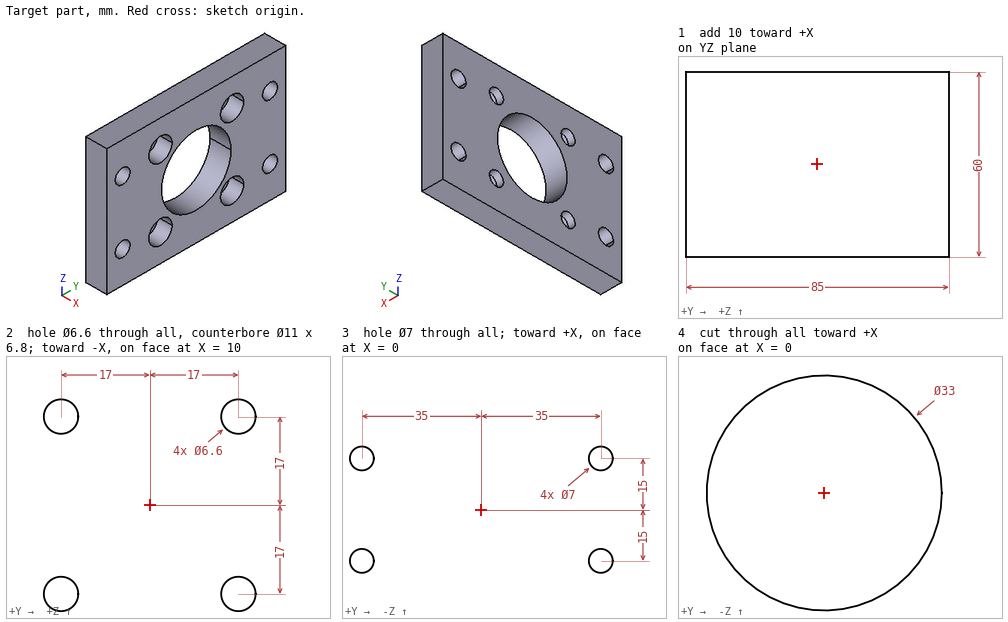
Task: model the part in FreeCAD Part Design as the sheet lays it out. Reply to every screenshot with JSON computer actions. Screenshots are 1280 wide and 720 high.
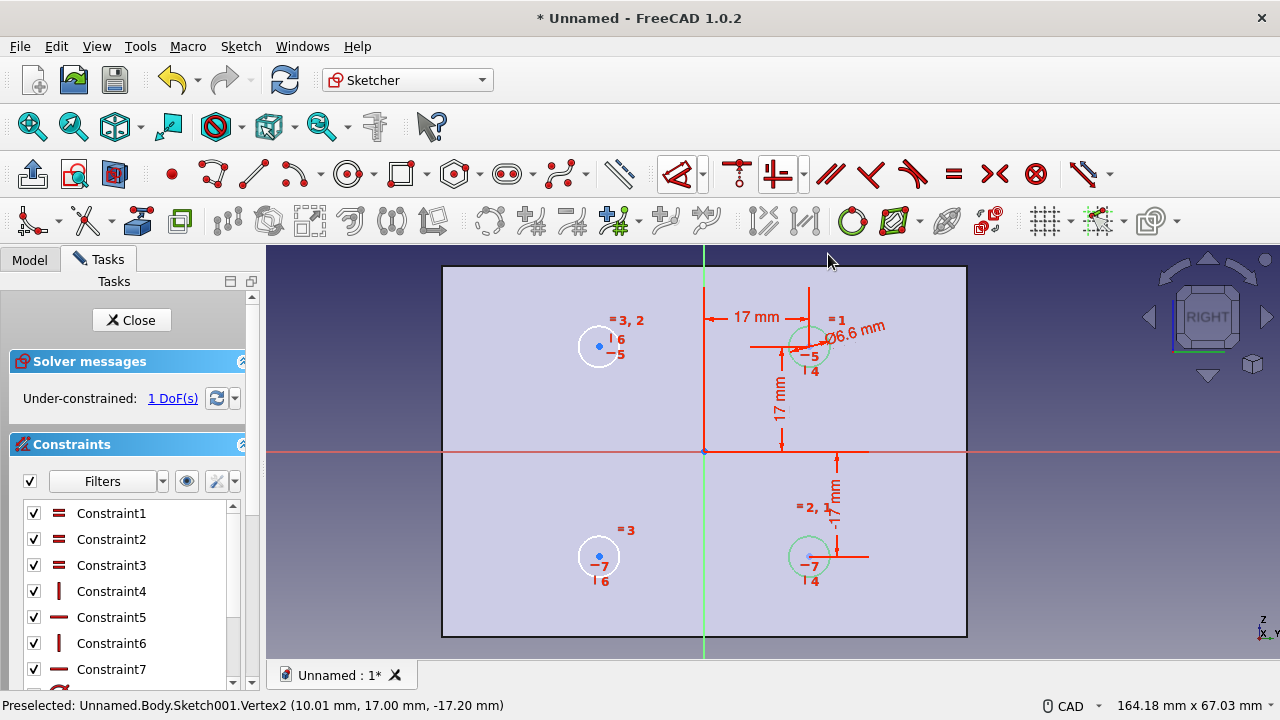
{"action": "left_click", "coordinate": [599, 347]}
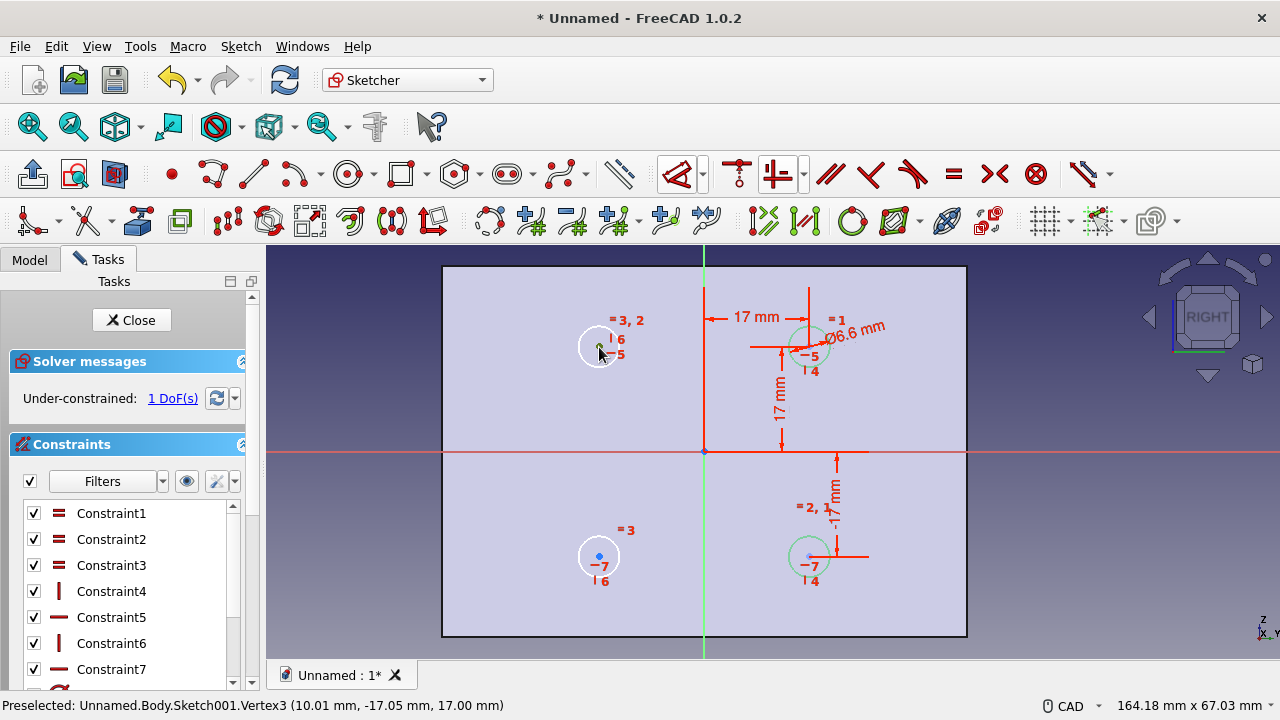
{"action": "key", "text": "l"}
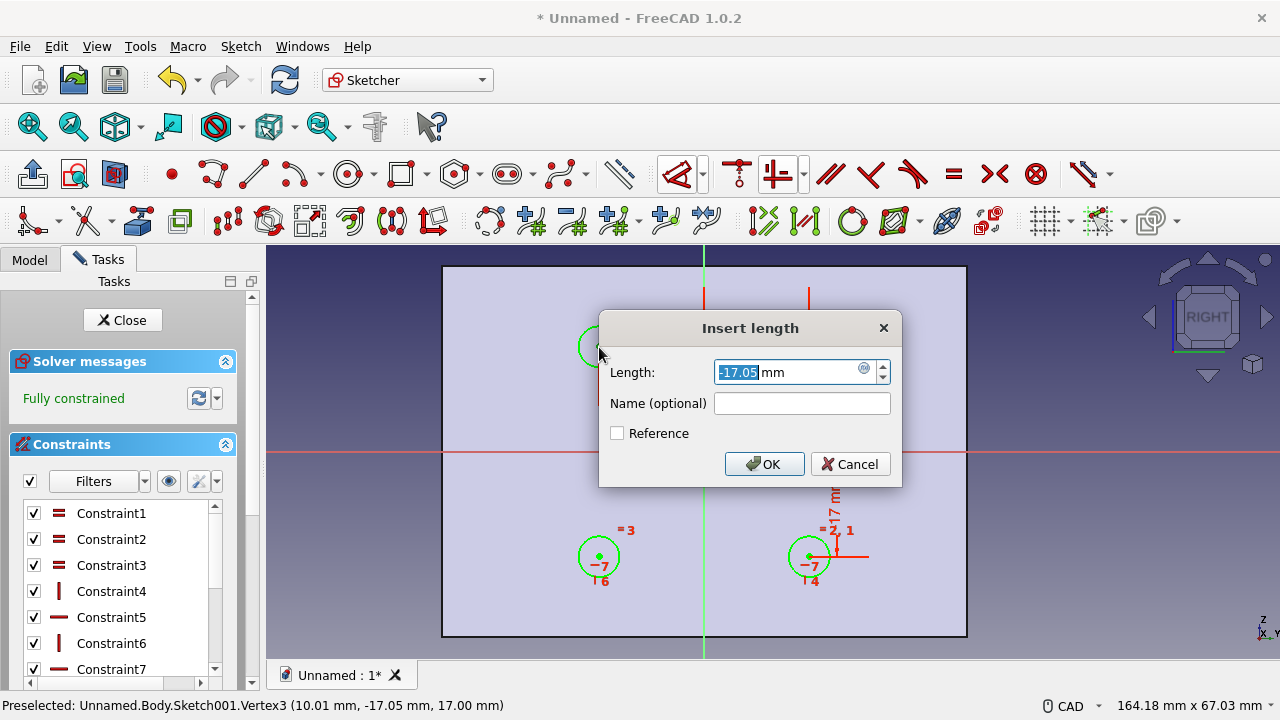
{"action": "type", "text": "-17"}
{"action": "key", "text": "Return"}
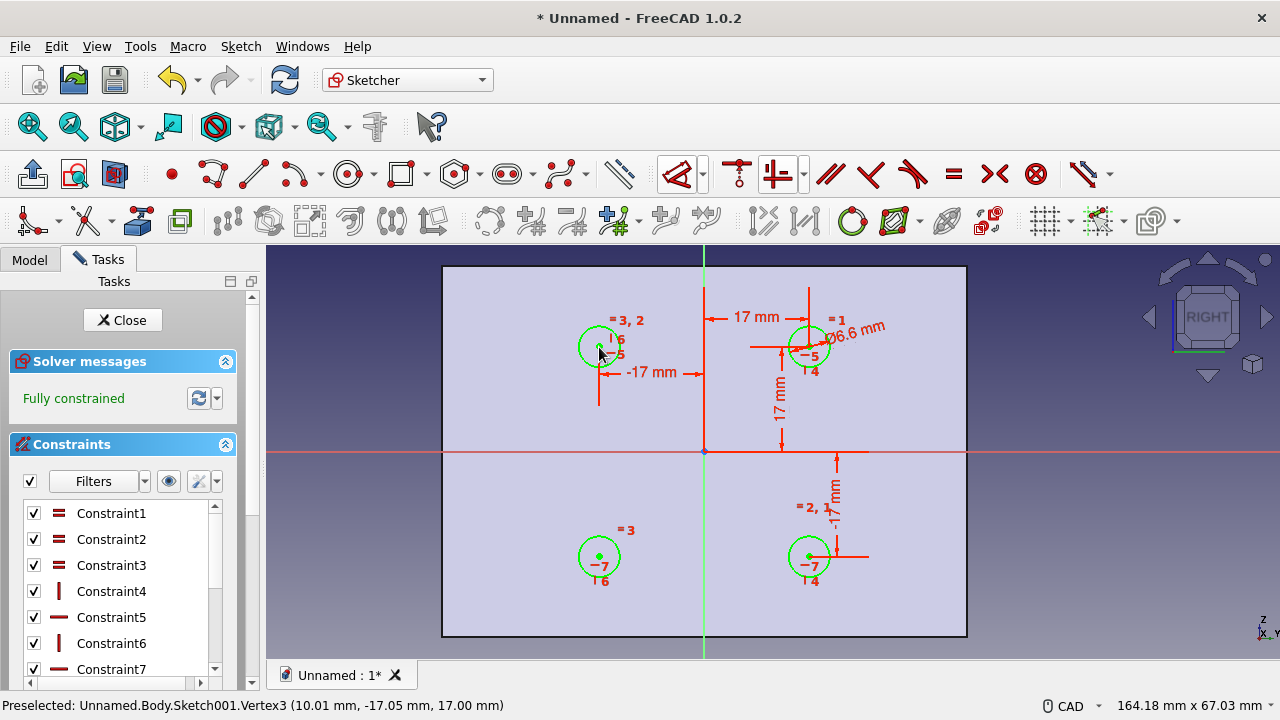
{"action": "left_click", "coordinate": [123, 320]}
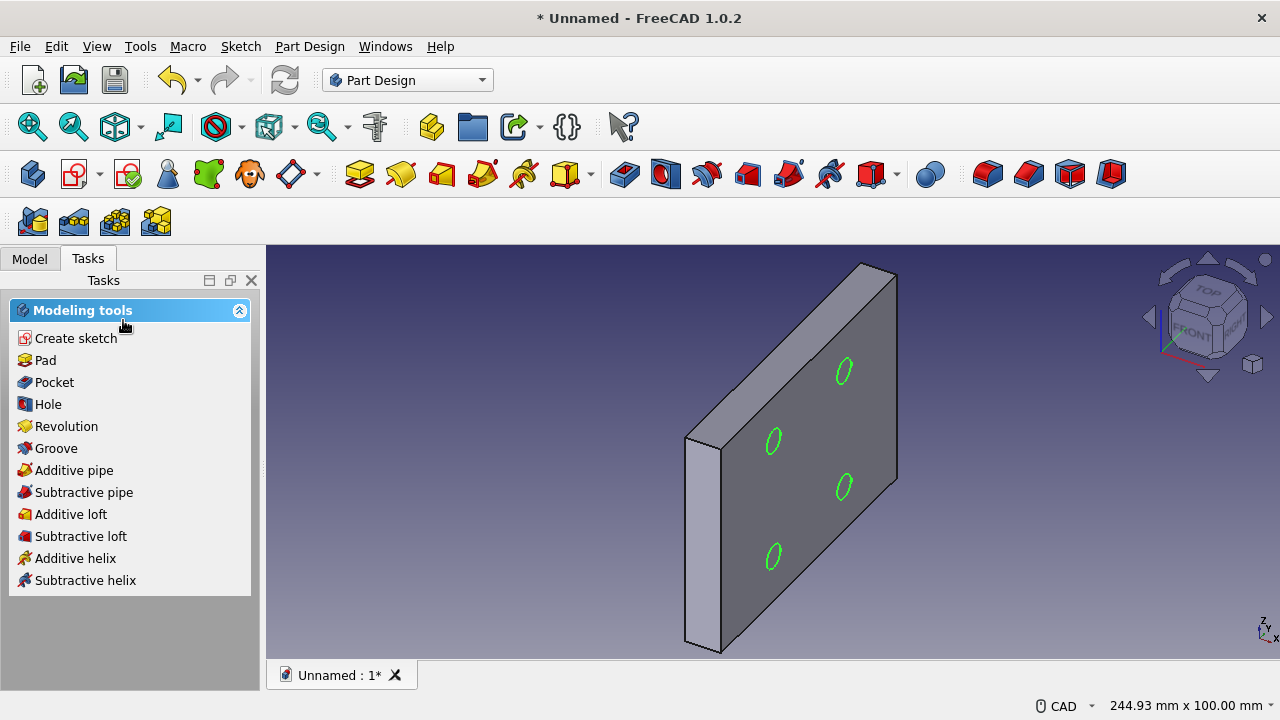
{"action": "left_click", "coordinate": [666, 174]}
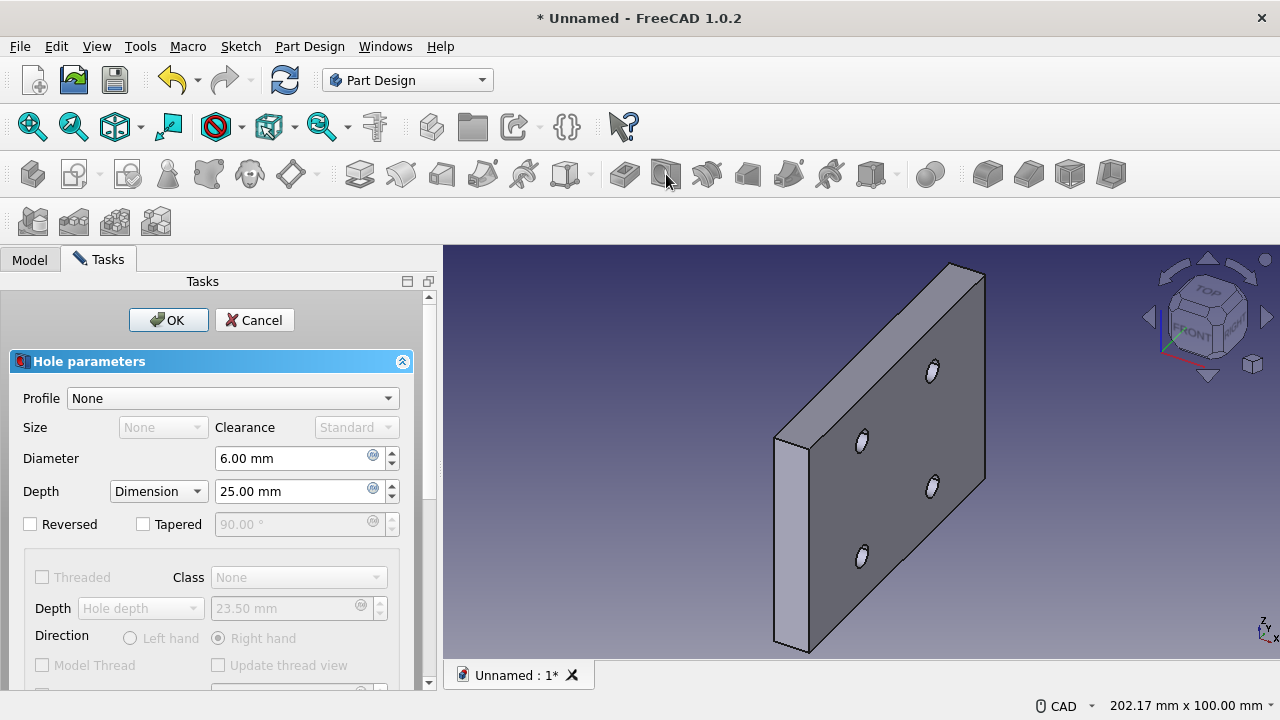
{"action": "triple_click", "coordinate": [300, 458]}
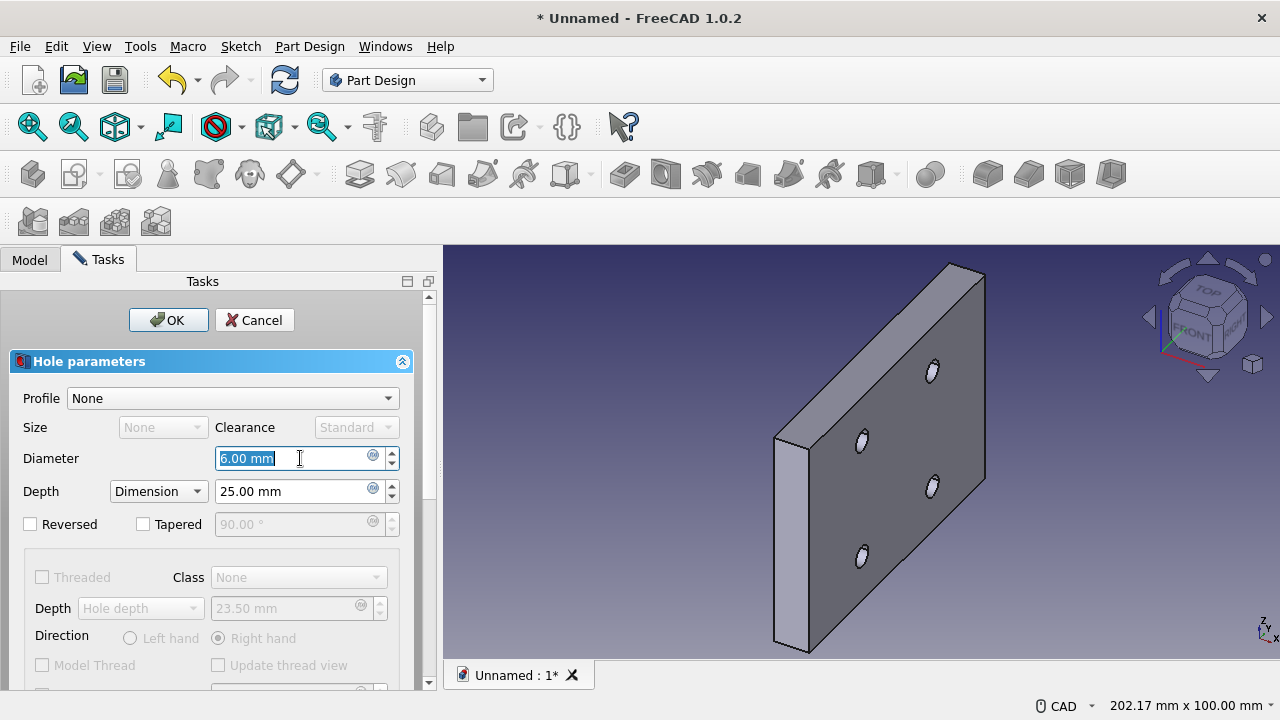
{"action": "type", "text": "6.6"}
{"action": "key", "text": "Tab"}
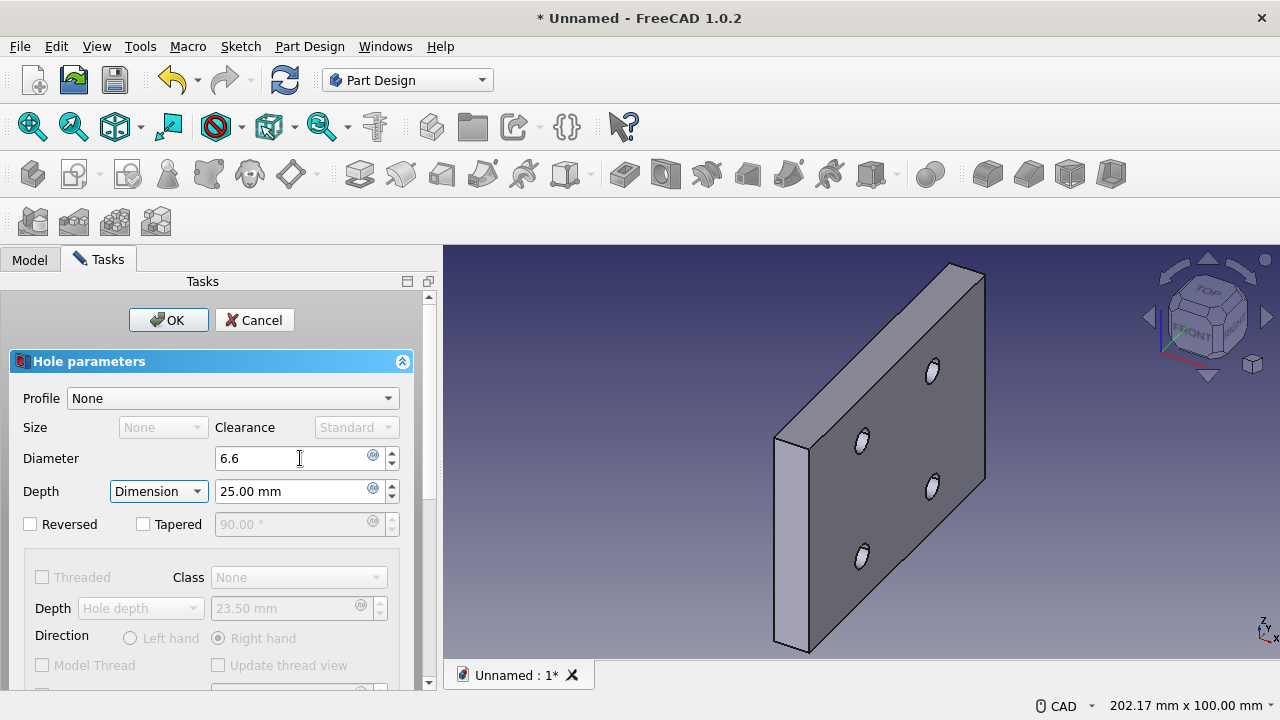
{"action": "left_click", "coordinate": [160, 492]}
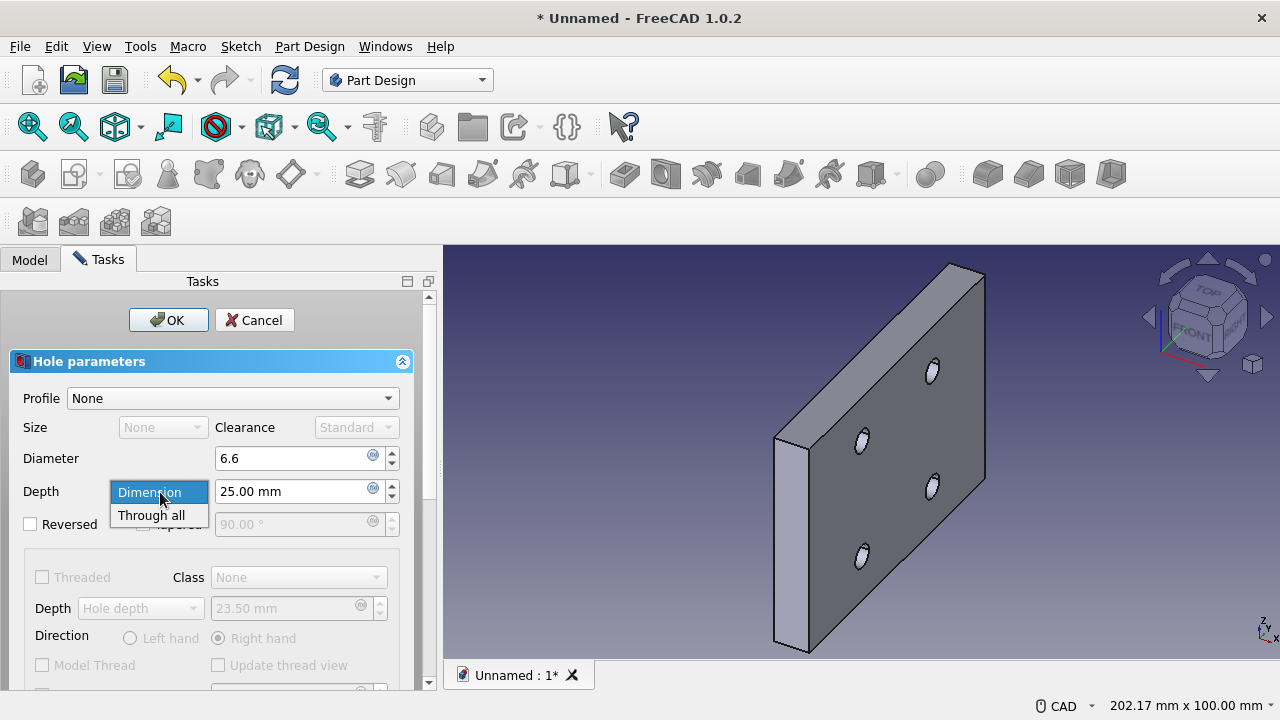
{"action": "left_click", "coordinate": [158, 516]}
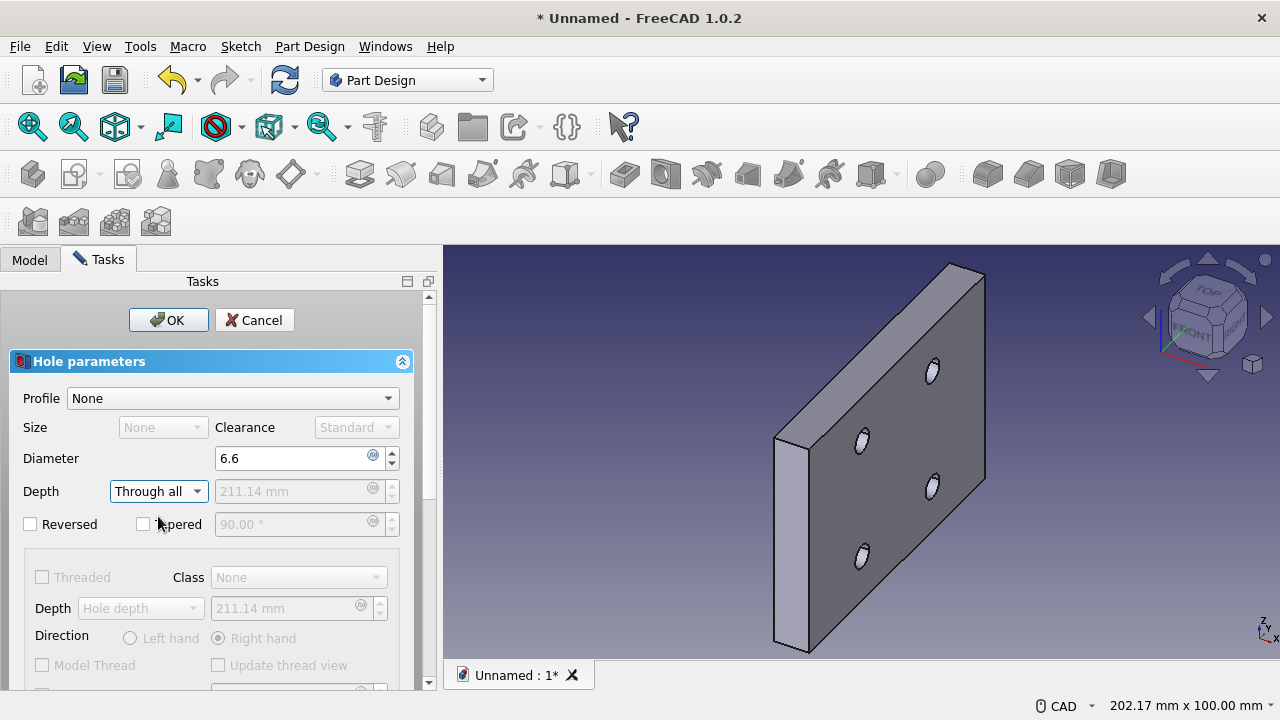
{"action": "scroll", "coordinate": [429, 490], "scroll_direction": "down", "scroll_amount": 3}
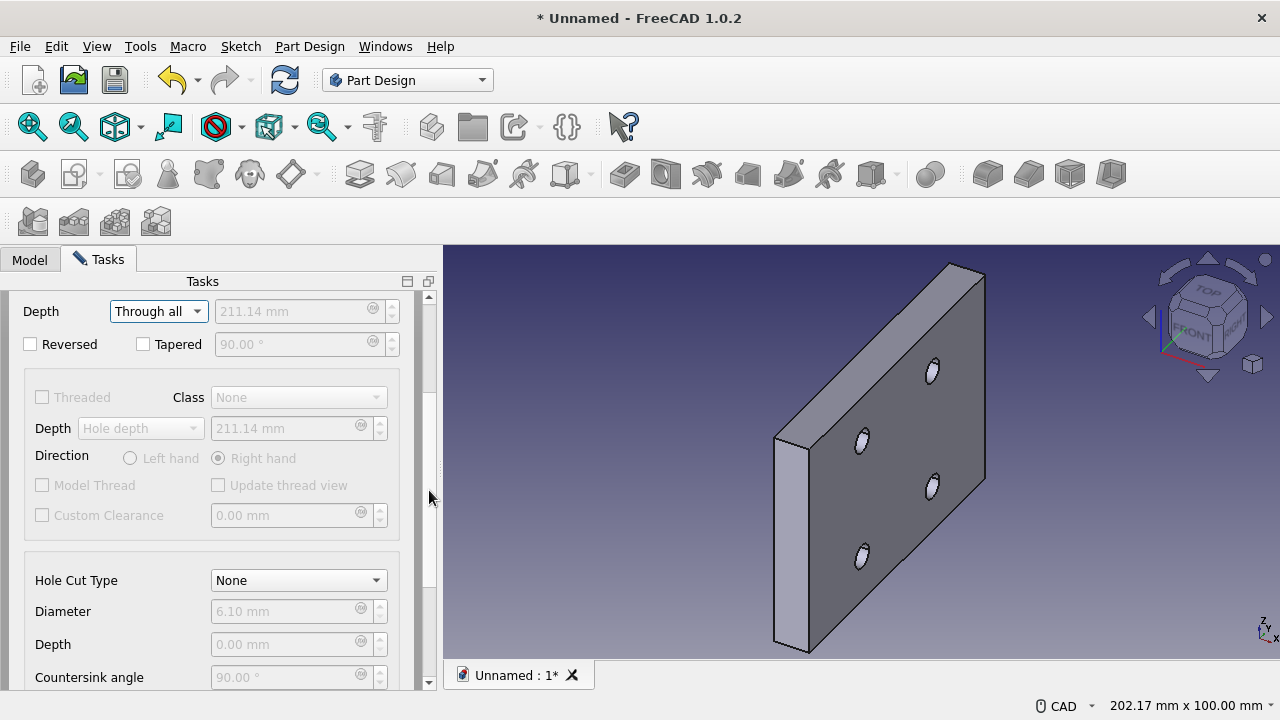
{"action": "left_click", "coordinate": [300, 580]}